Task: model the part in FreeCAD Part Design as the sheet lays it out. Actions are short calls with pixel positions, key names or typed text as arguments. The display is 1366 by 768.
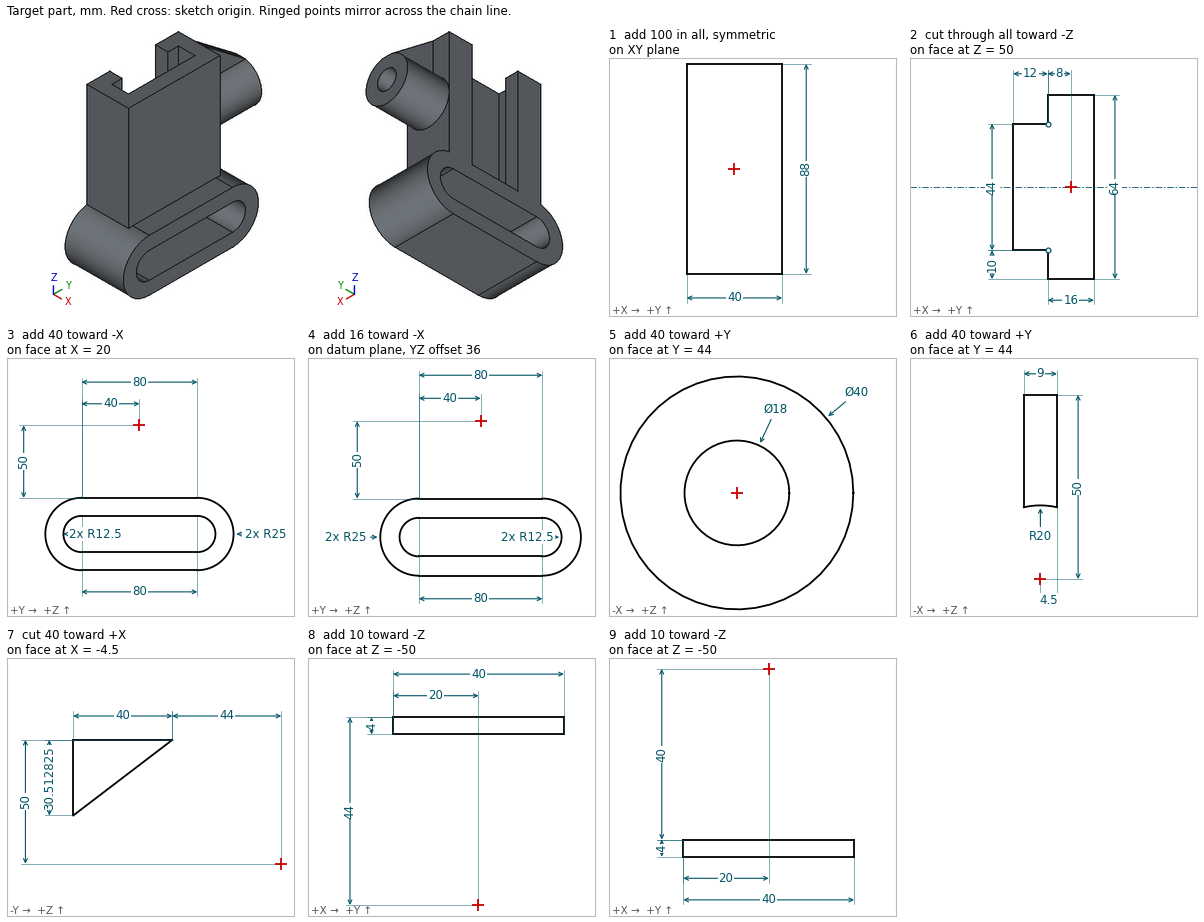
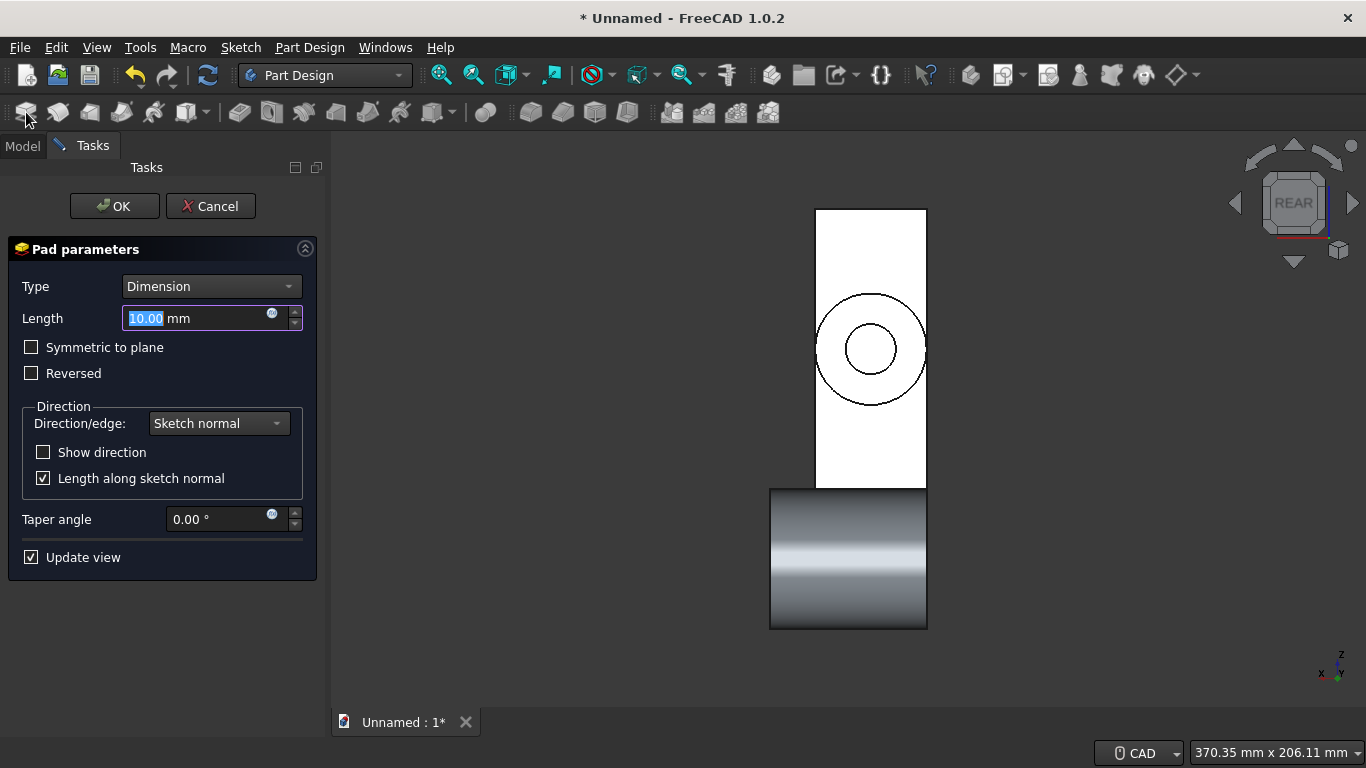
text(40)
key(Tab)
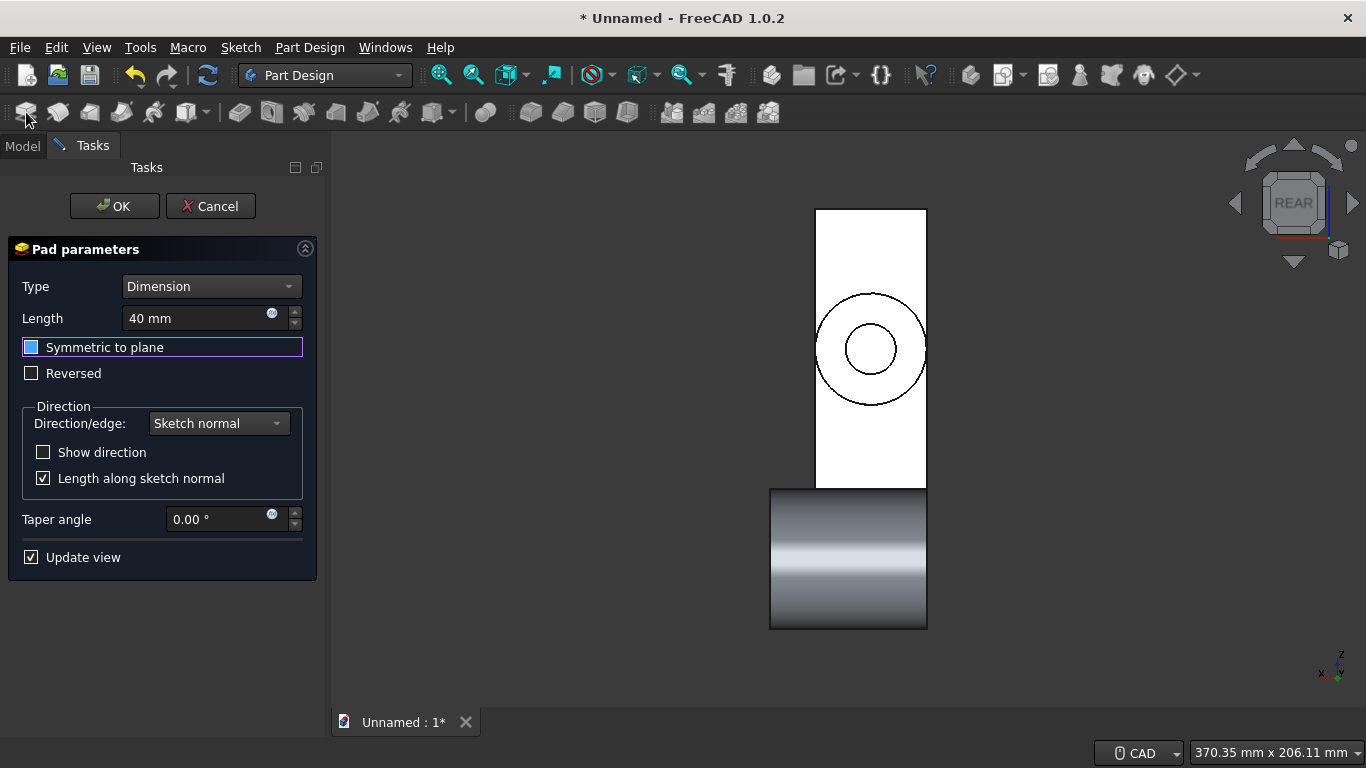
click(115, 206)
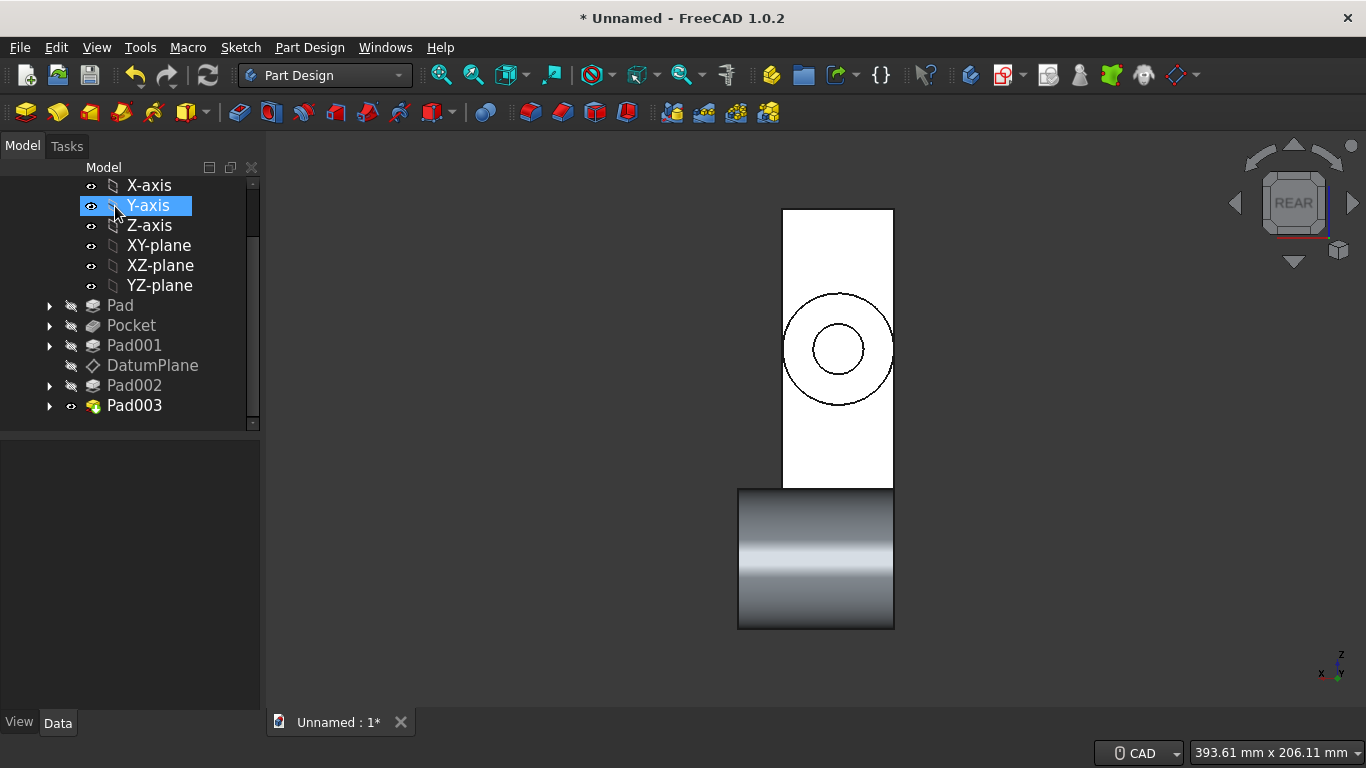
click(854, 438)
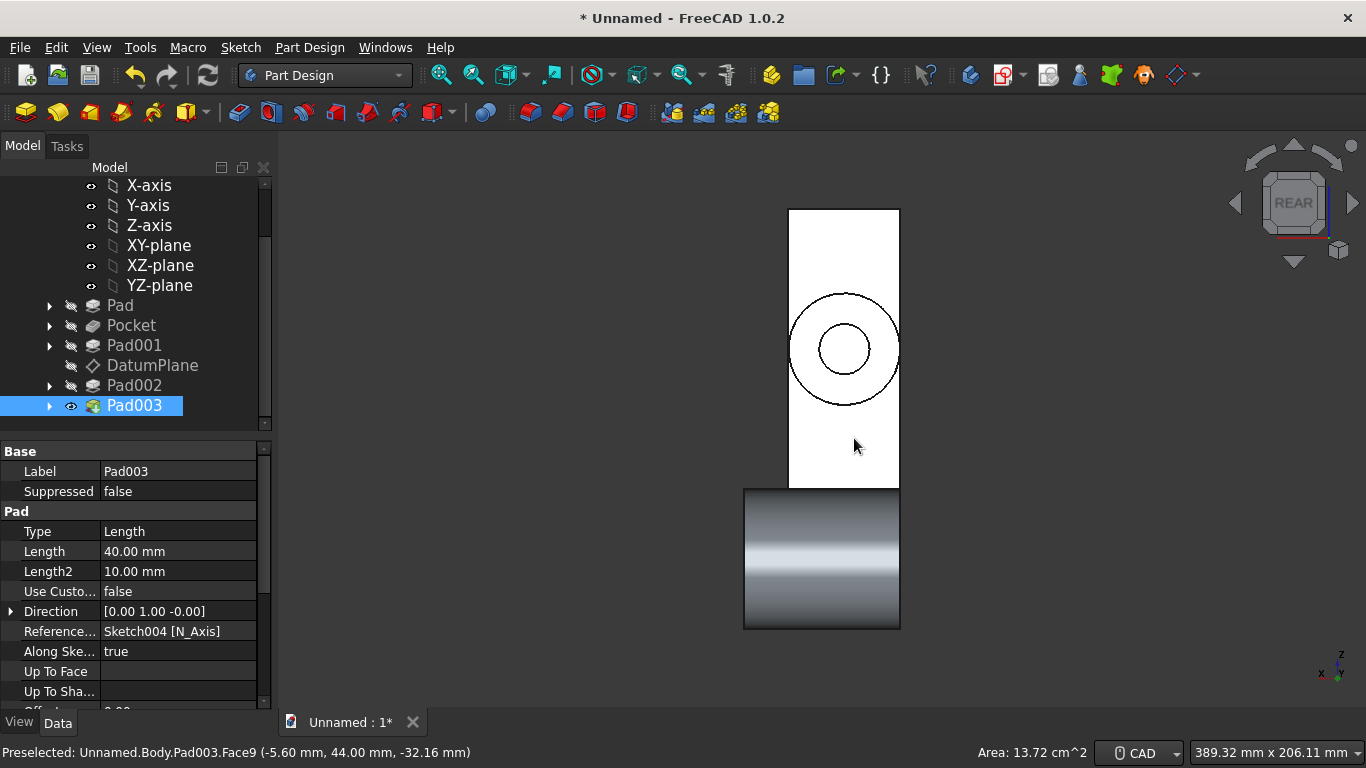
click(1004, 76)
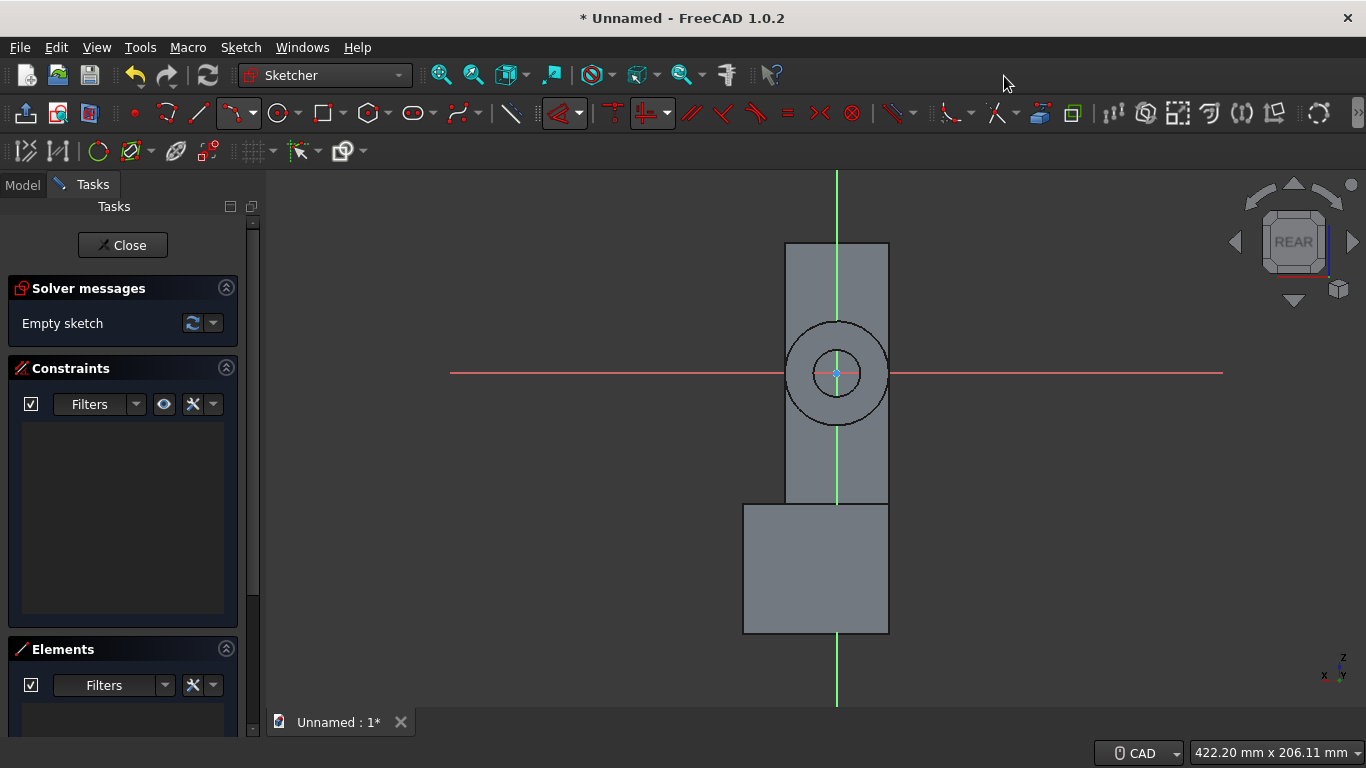
click(90, 114)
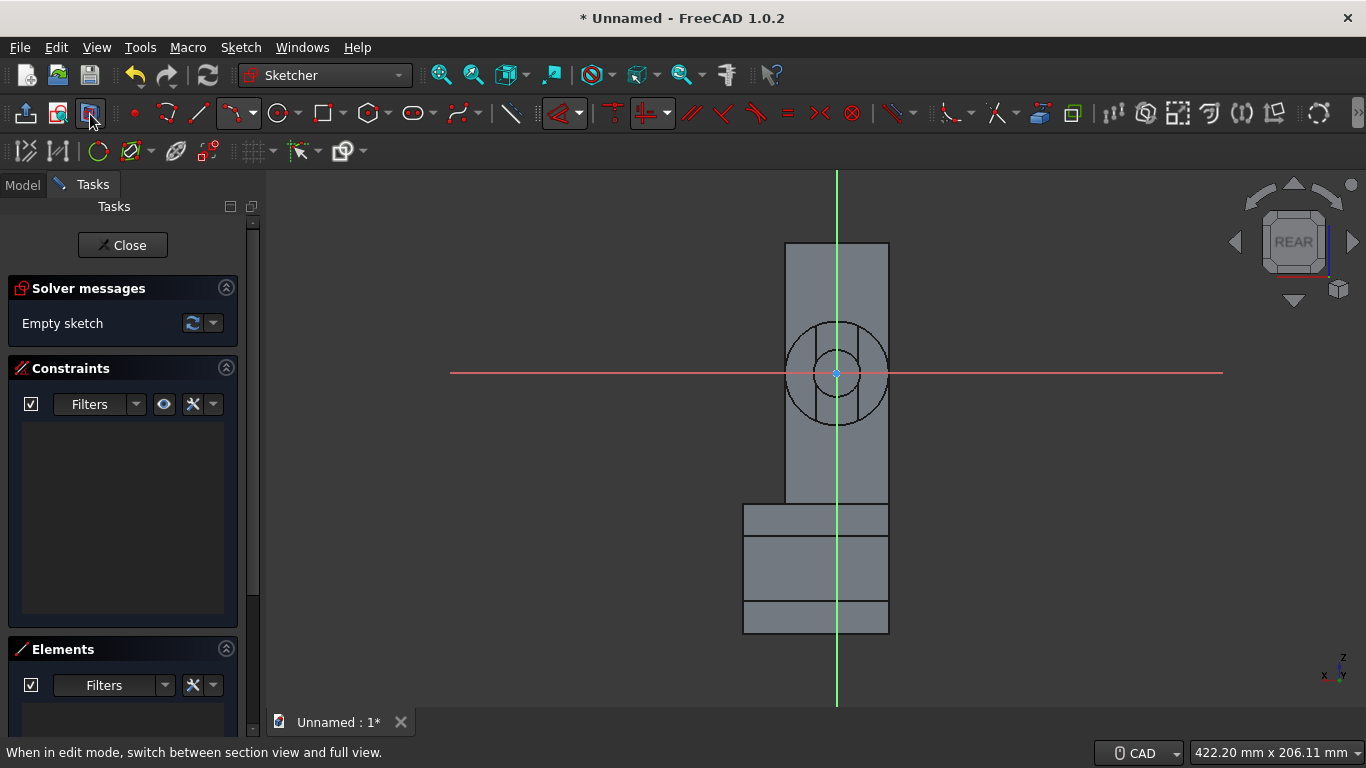
scroll(889, 232, up, 5)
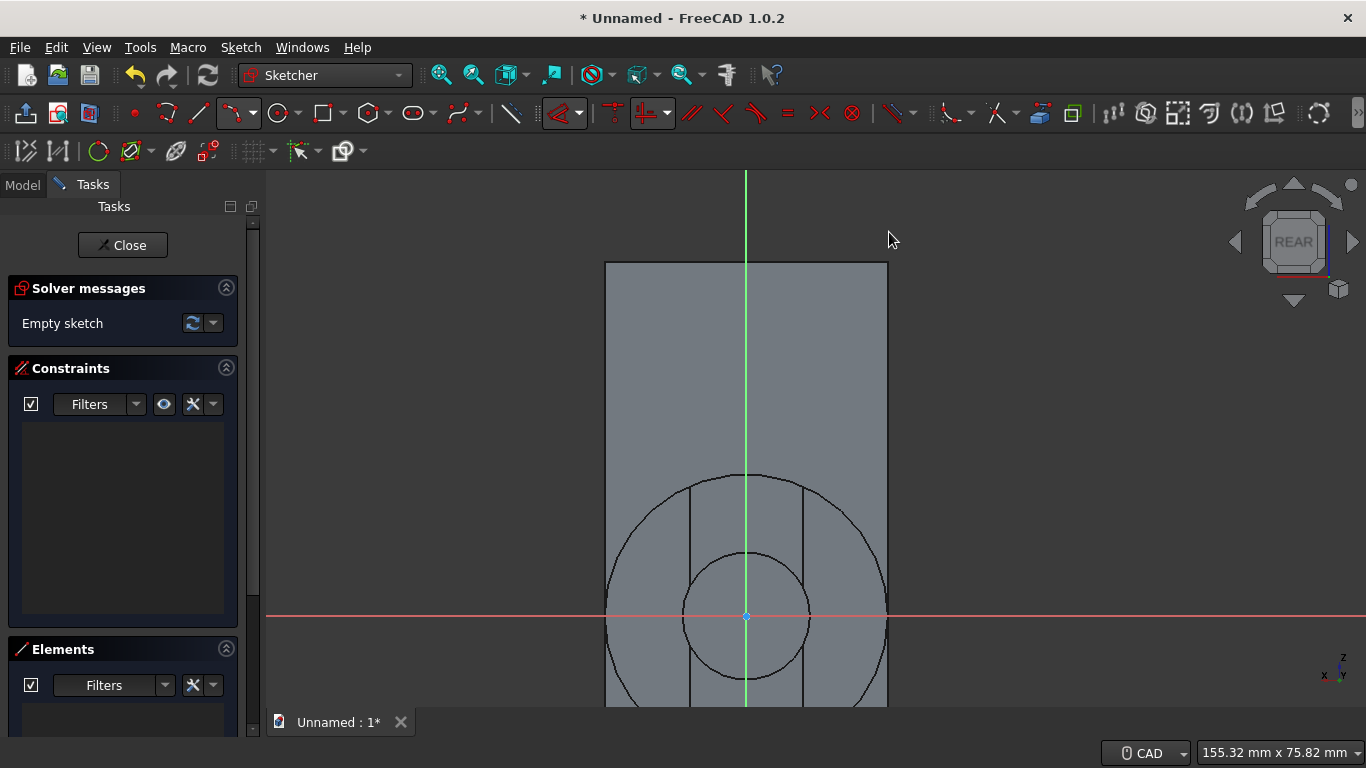
key(g)
key(m)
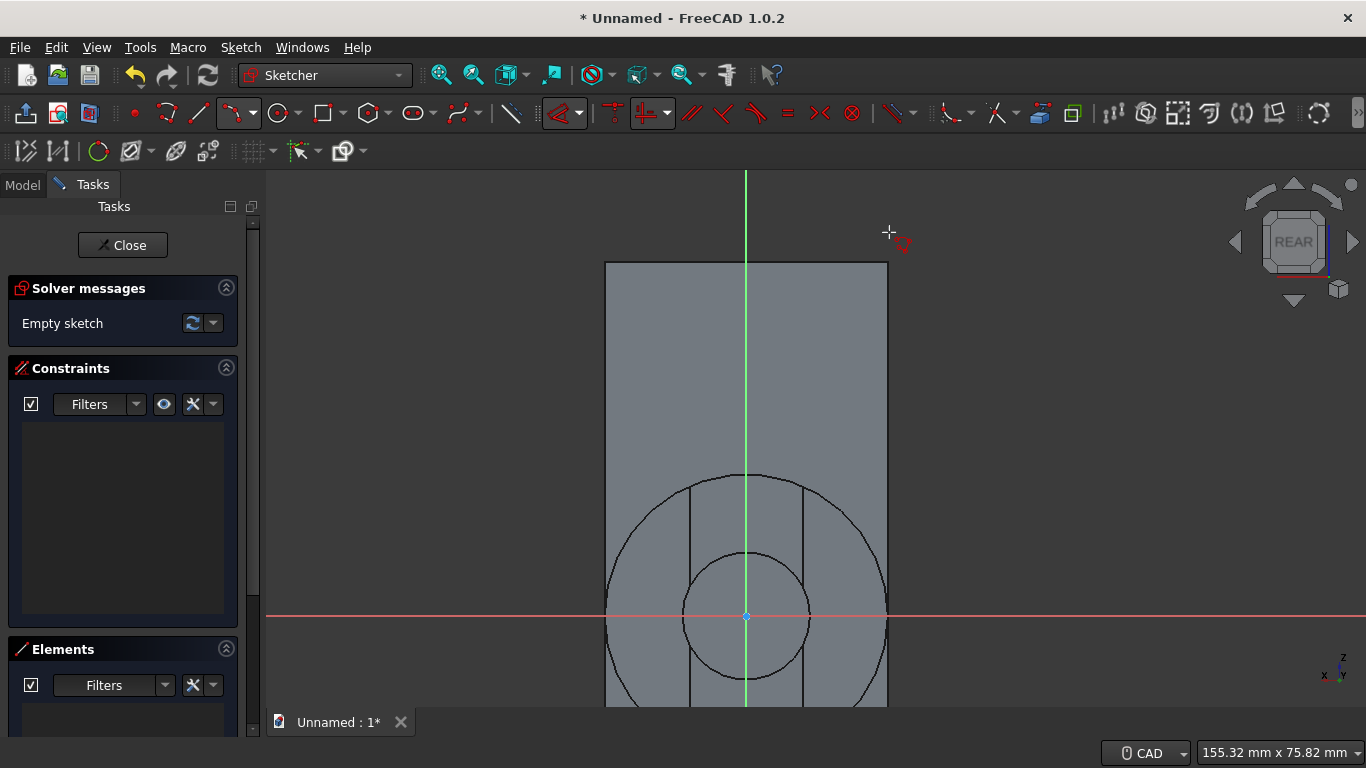
click(778, 478)
click(778, 262)
click(714, 262)
click(714, 478)
right_click(714, 478)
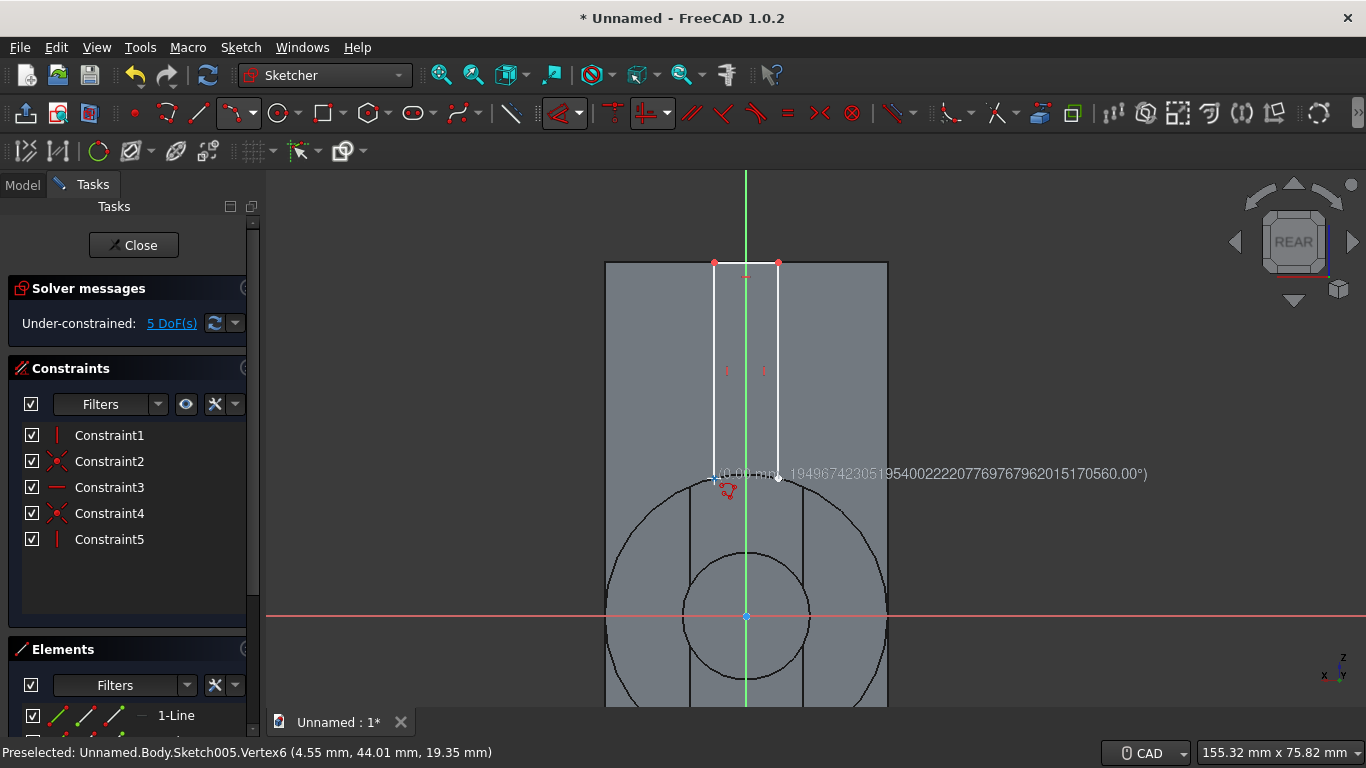
key(g)
key(3)
key(a)